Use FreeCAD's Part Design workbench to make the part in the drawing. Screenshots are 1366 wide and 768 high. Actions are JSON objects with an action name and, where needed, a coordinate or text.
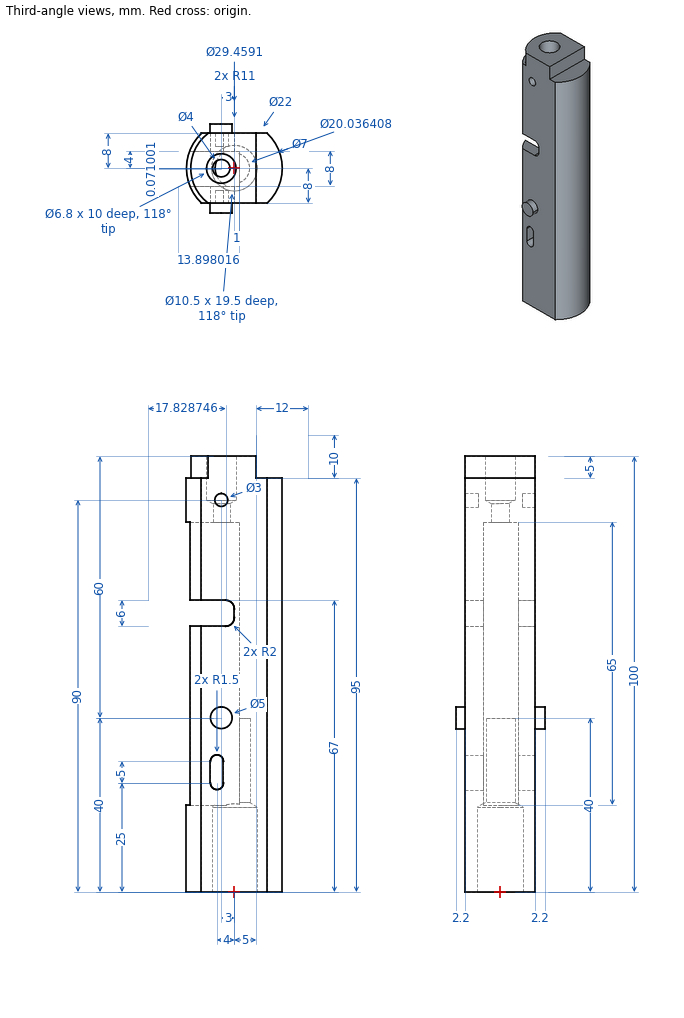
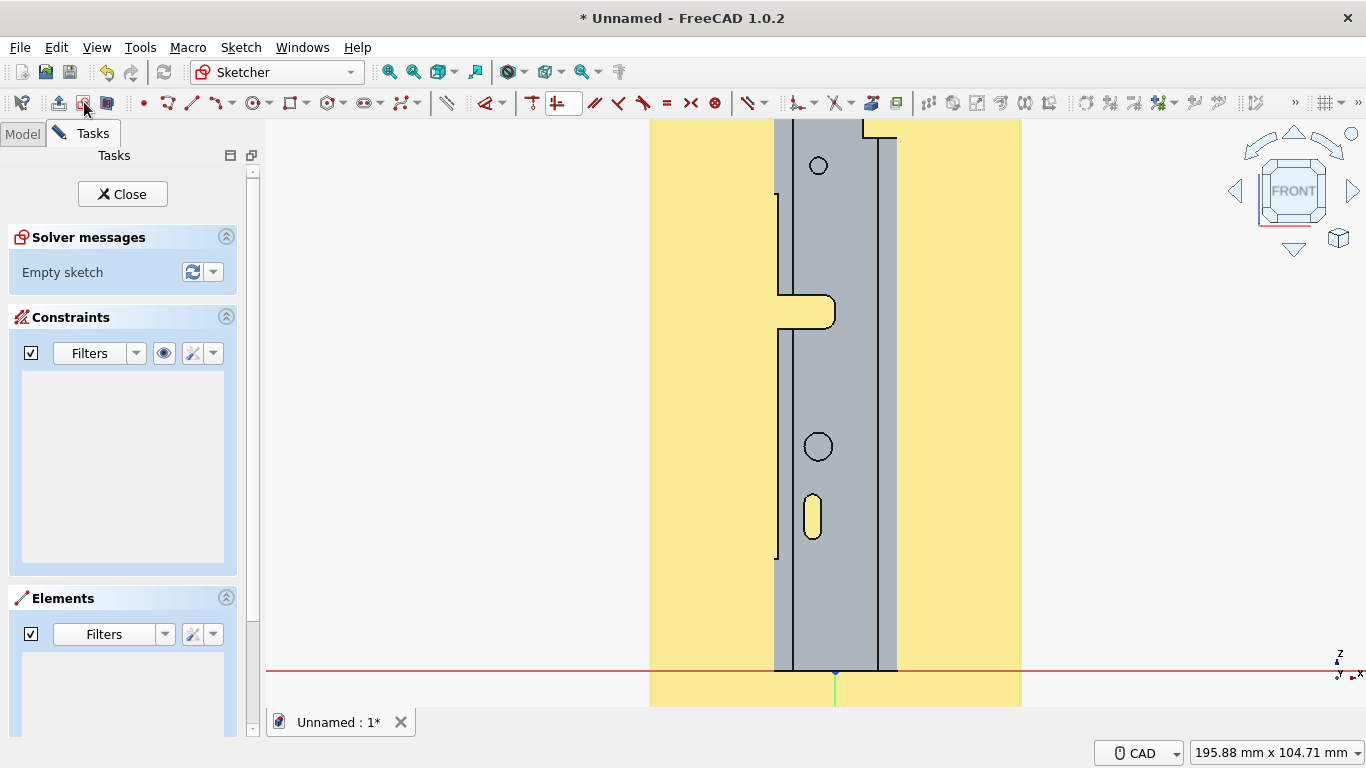
{"action": "key", "text": "q s"}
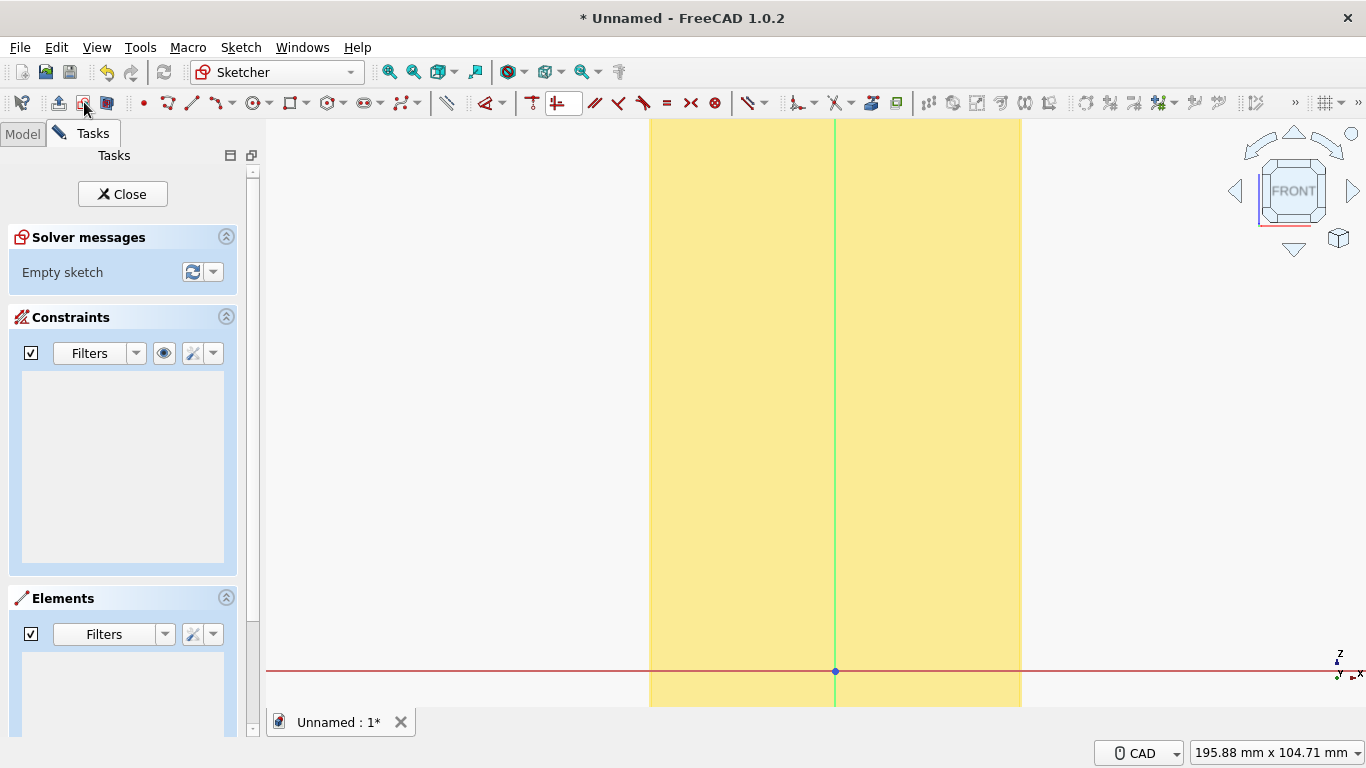
{"action": "scroll", "coordinate": [824, 449], "scroll_direction": "up", "scroll_amount": 13}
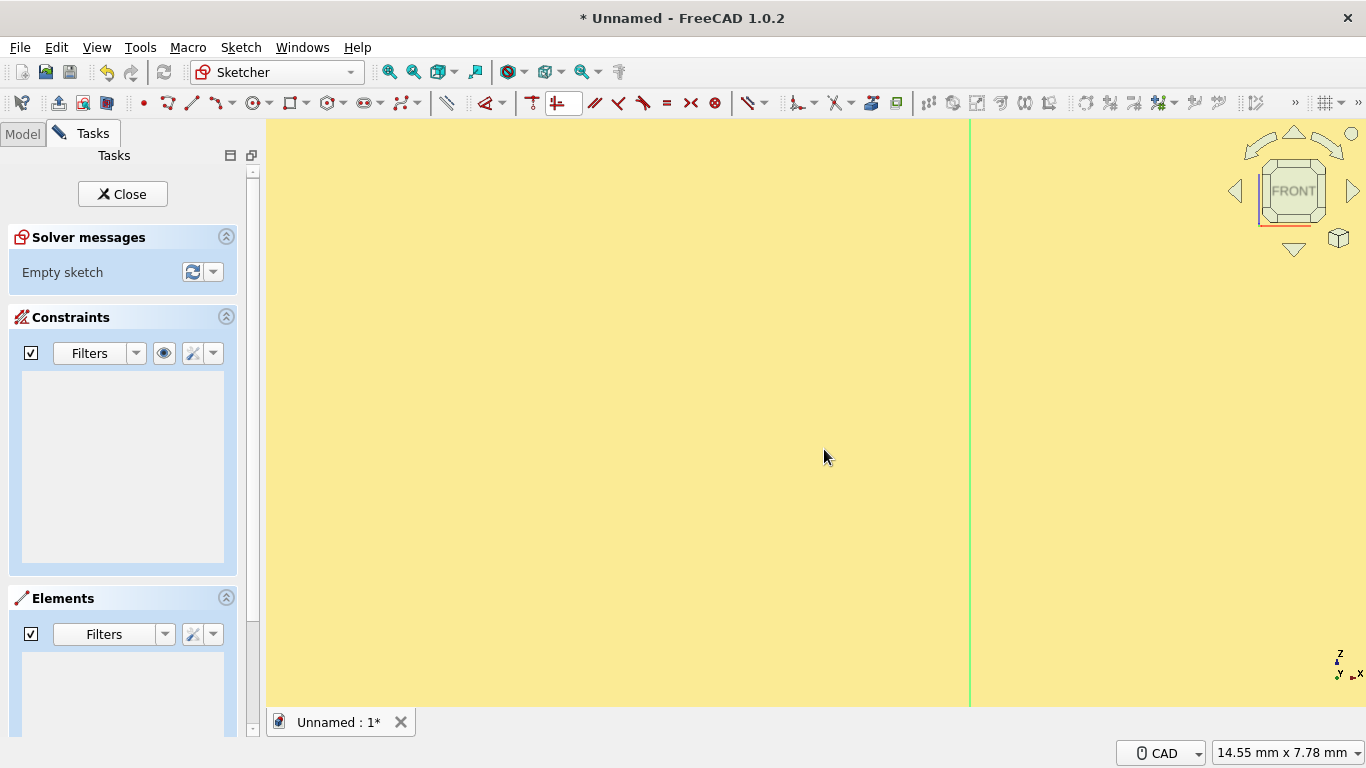
{"action": "key", "text": "g c"}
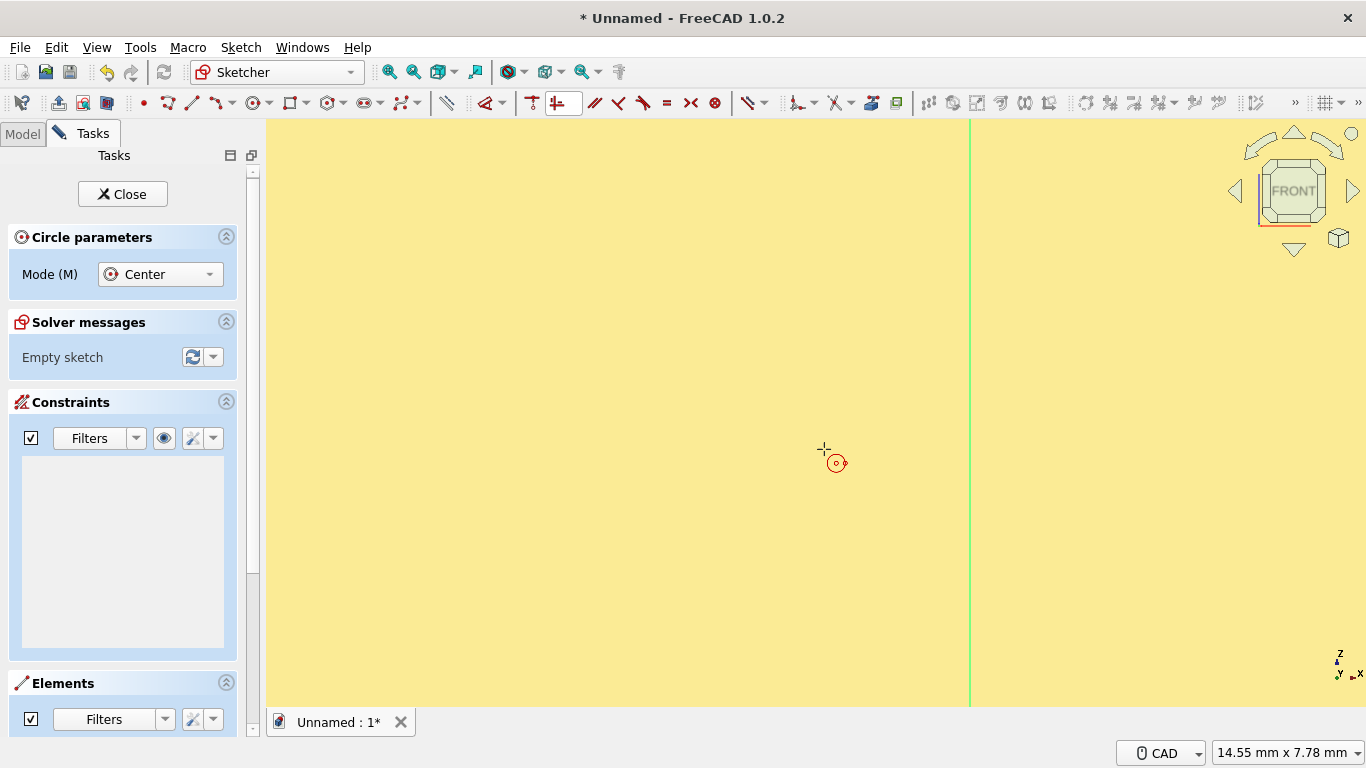
{"action": "left_click", "coordinate": [743, 410]}
{"action": "mouse_move", "coordinate": [877, 276]}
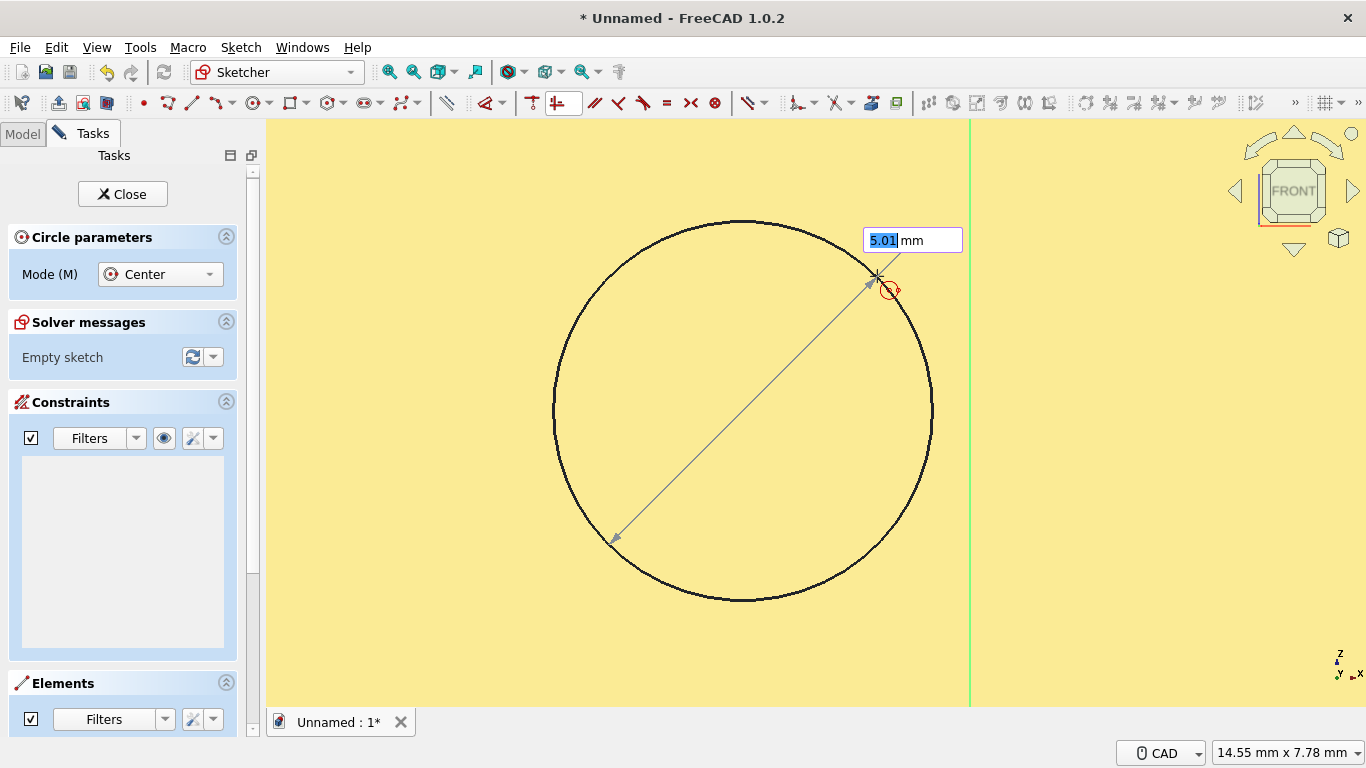
{"action": "type", "text": "5"}
{"action": "key", "text": "Return"}
{"action": "key", "text": "Escape"}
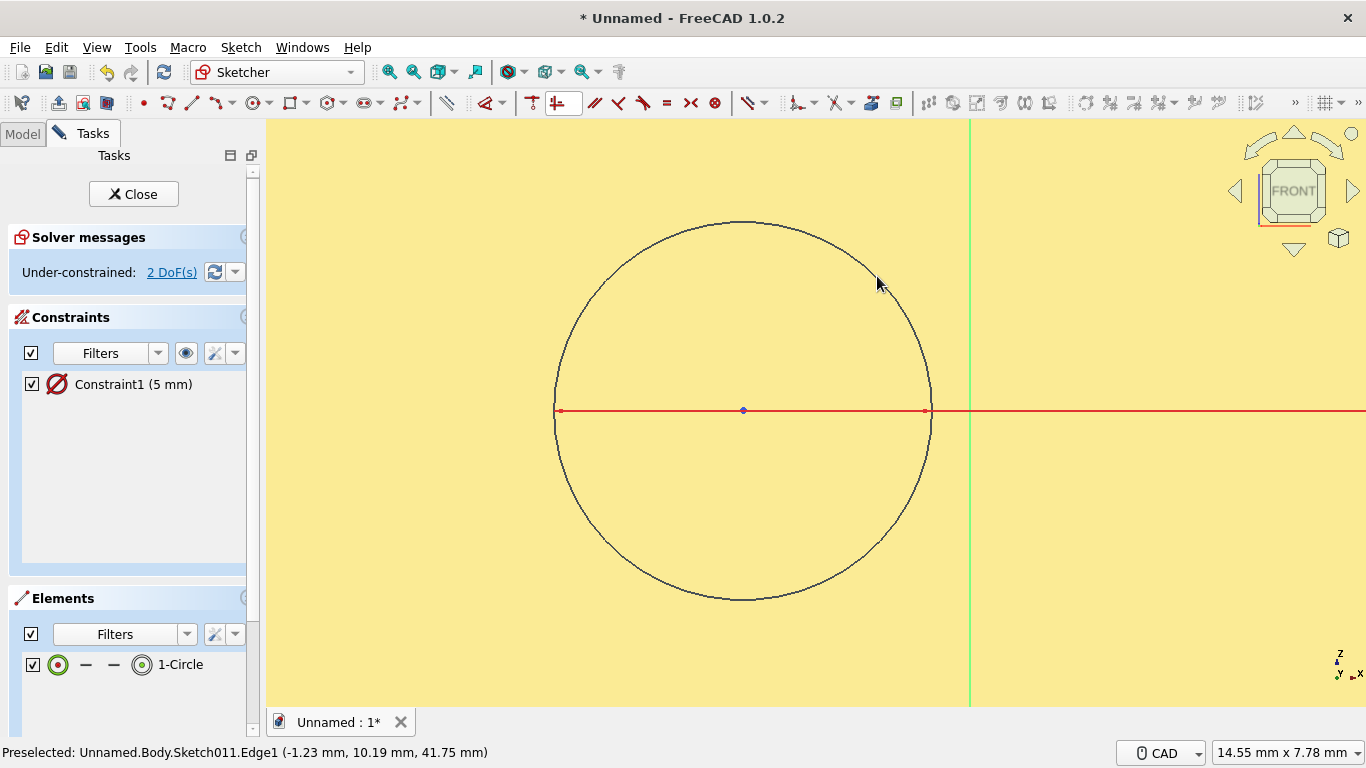
{"action": "key", "text": "d"}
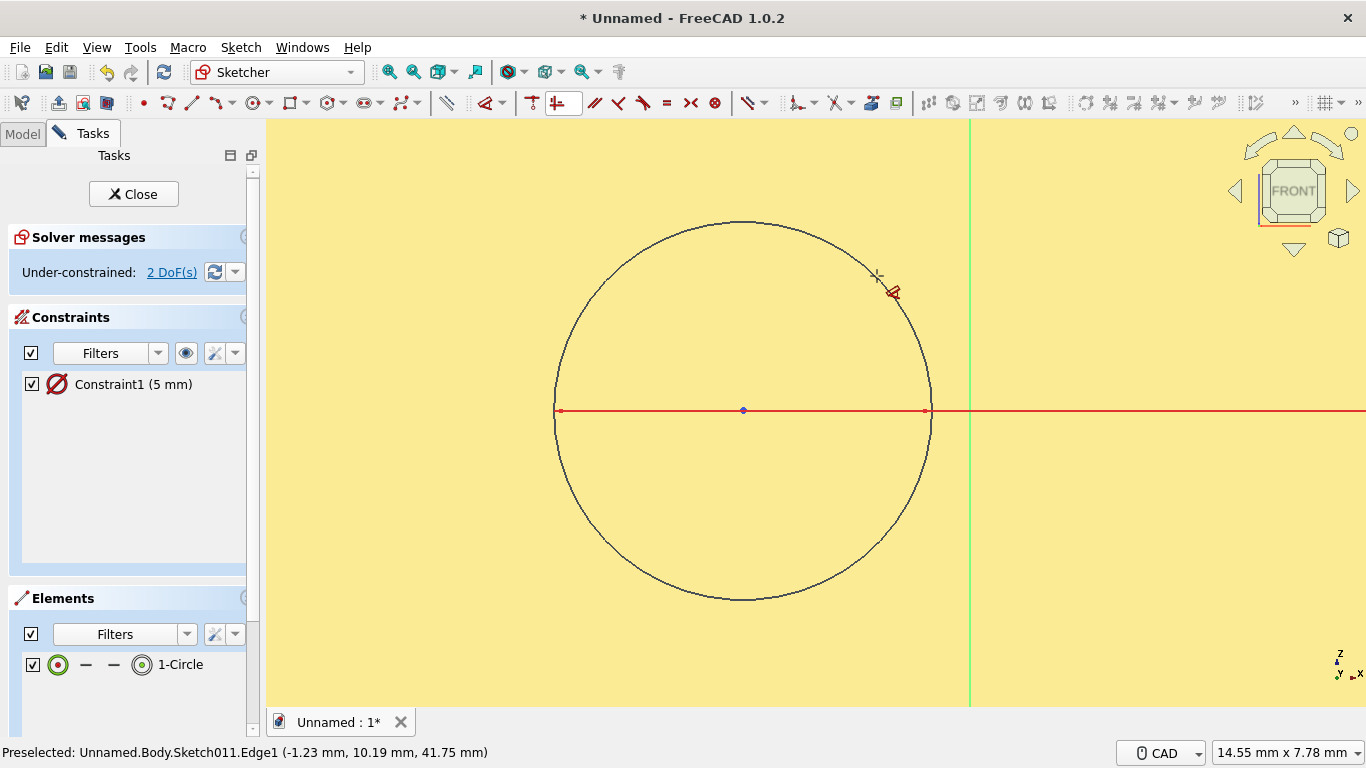
{"action": "left_click", "coordinate": [743, 411]}
{"action": "left_click", "coordinate": [856, 377]}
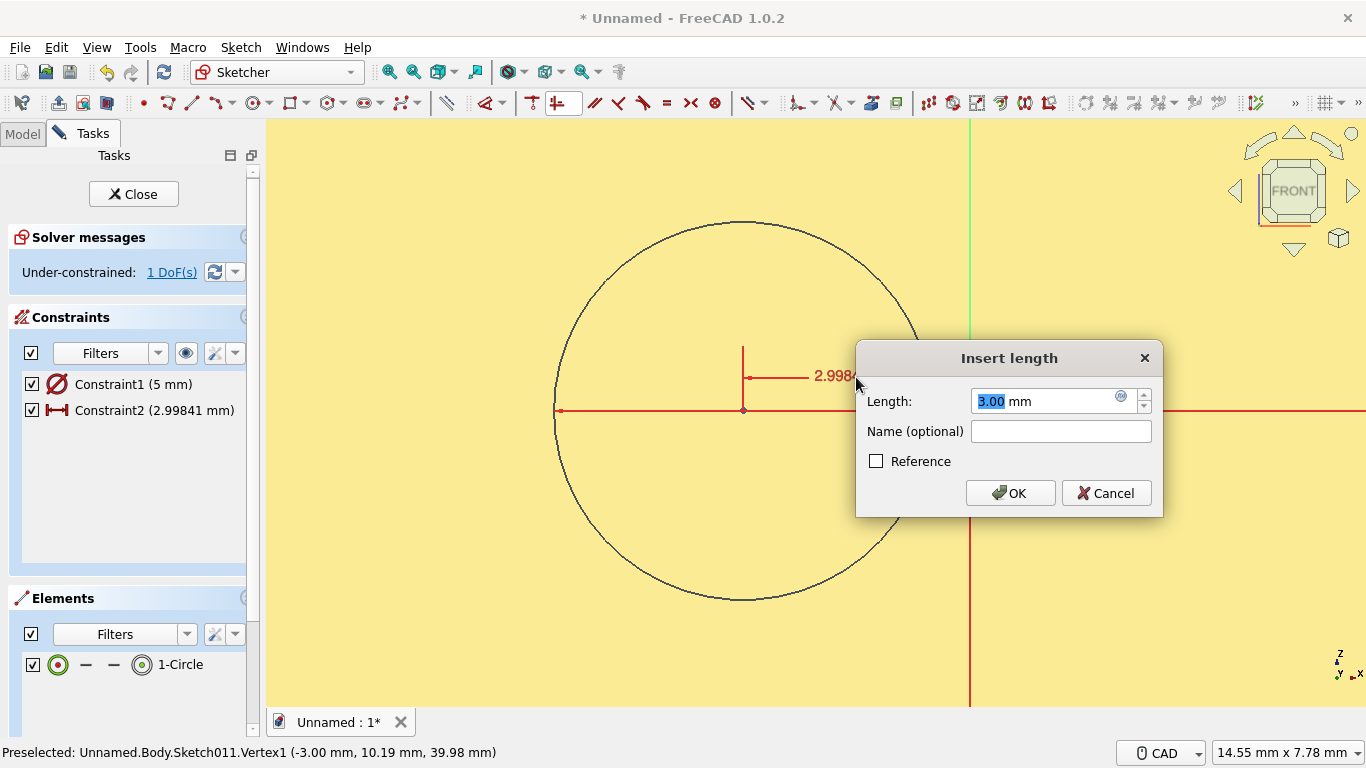
{"action": "type", "text": "3"}
{"action": "key", "text": "Return"}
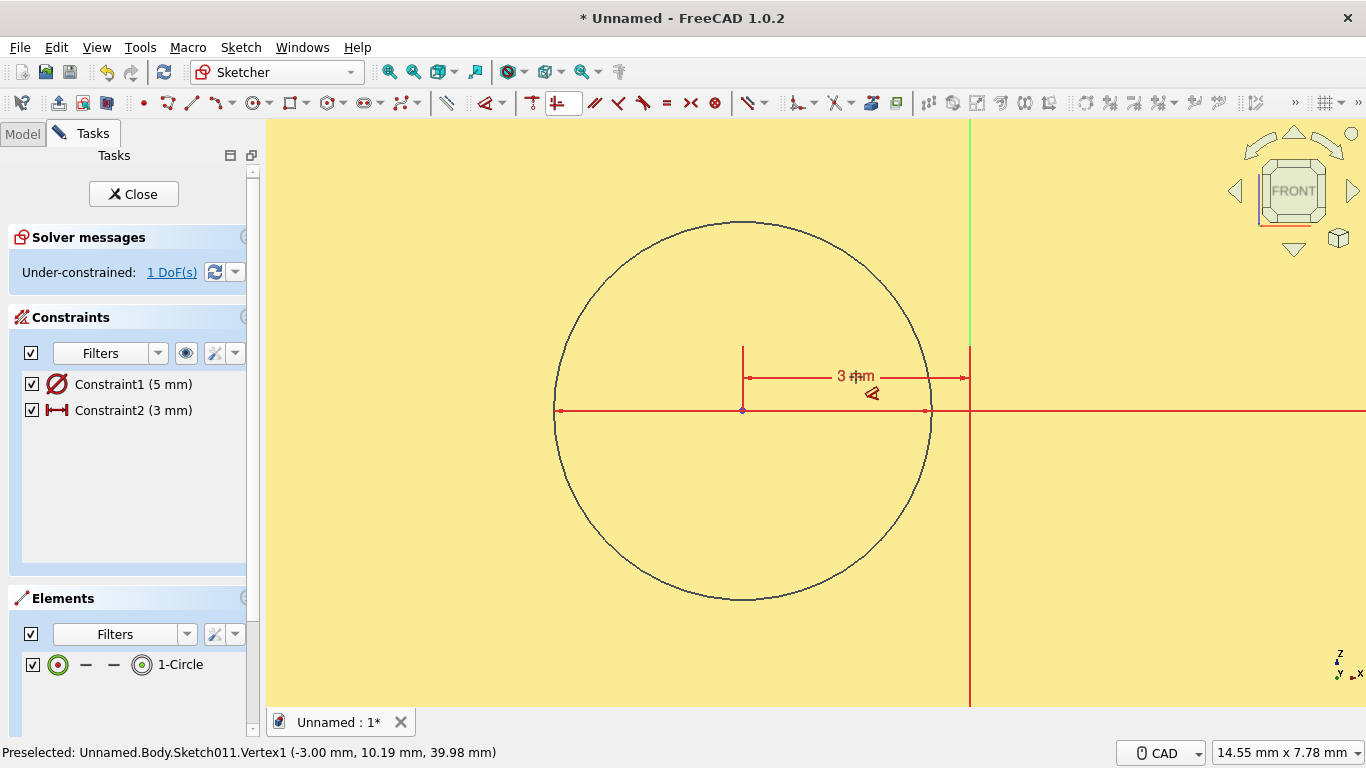
{"action": "left_click", "coordinate": [743, 411]}
{"action": "left_click", "coordinate": [1004, 545]}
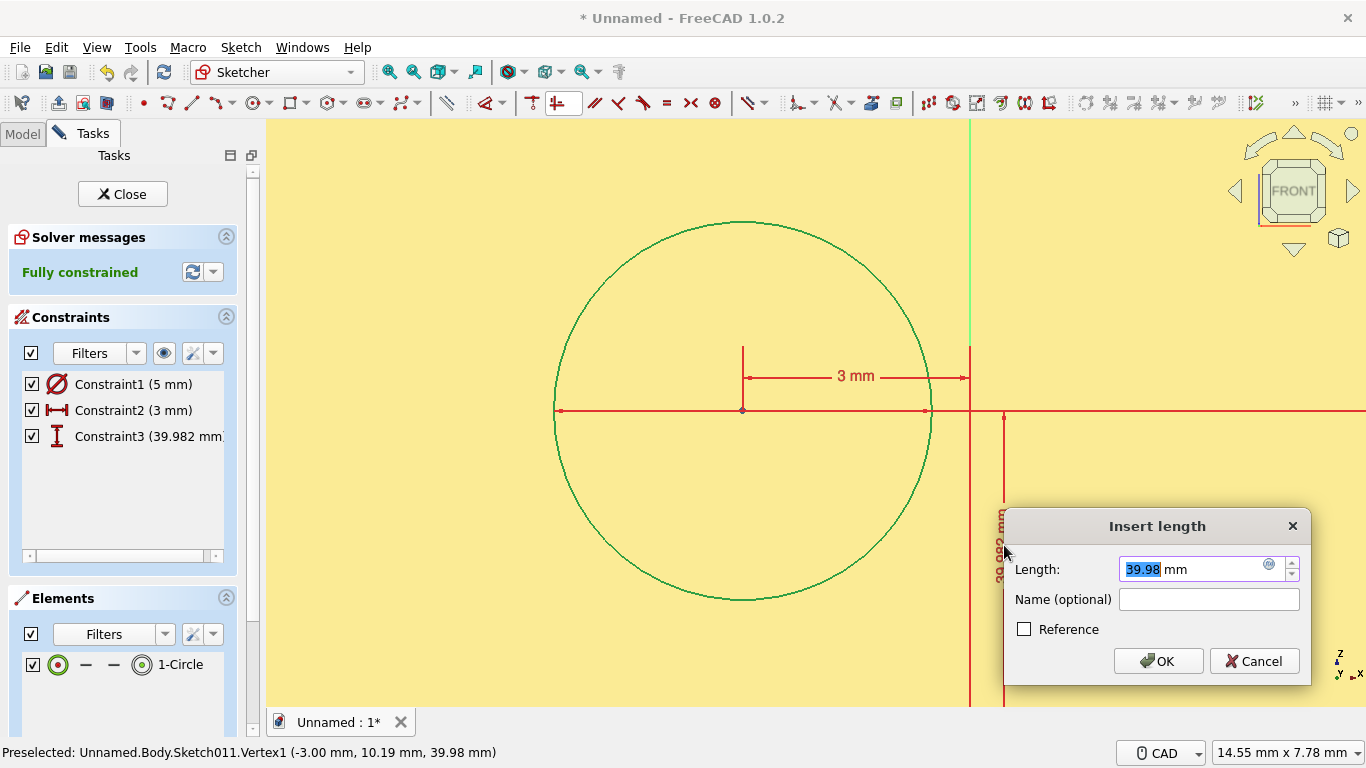
{"action": "type", "text": "40"}
{"action": "key", "text": "Return"}
{"action": "key", "text": "Escape"}